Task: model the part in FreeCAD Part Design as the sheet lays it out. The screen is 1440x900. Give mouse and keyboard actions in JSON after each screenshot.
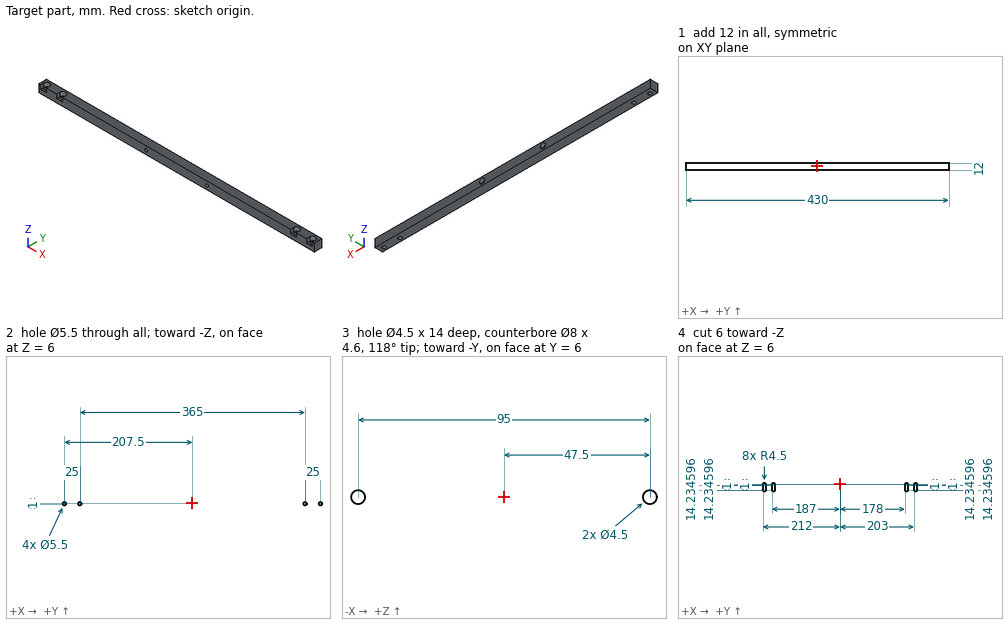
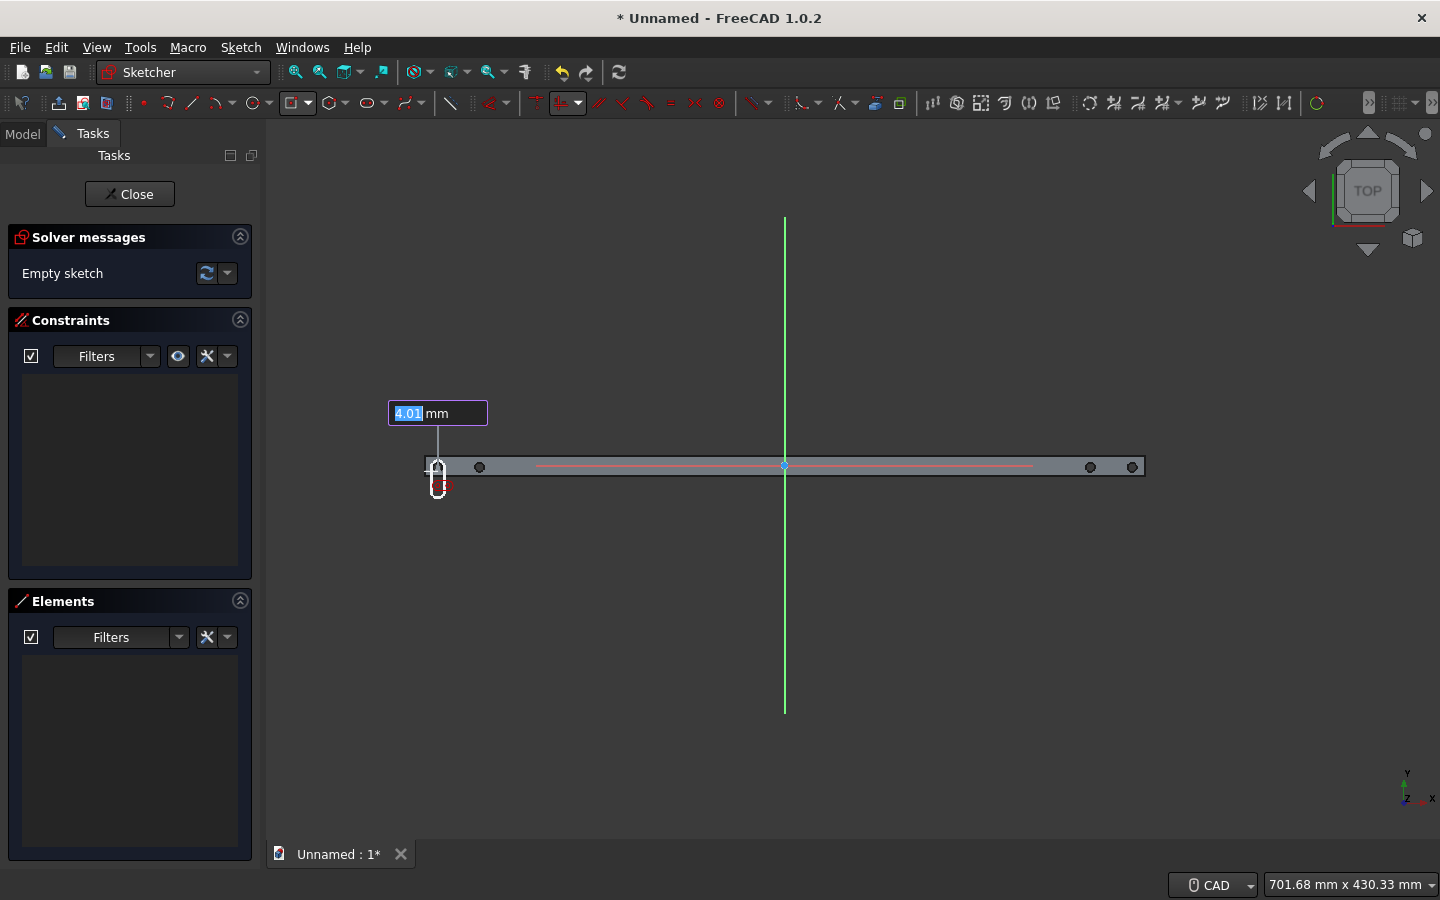
{"action": "scroll", "coordinate": [445, 479], "scroll_direction": "up", "scroll_amount": 4}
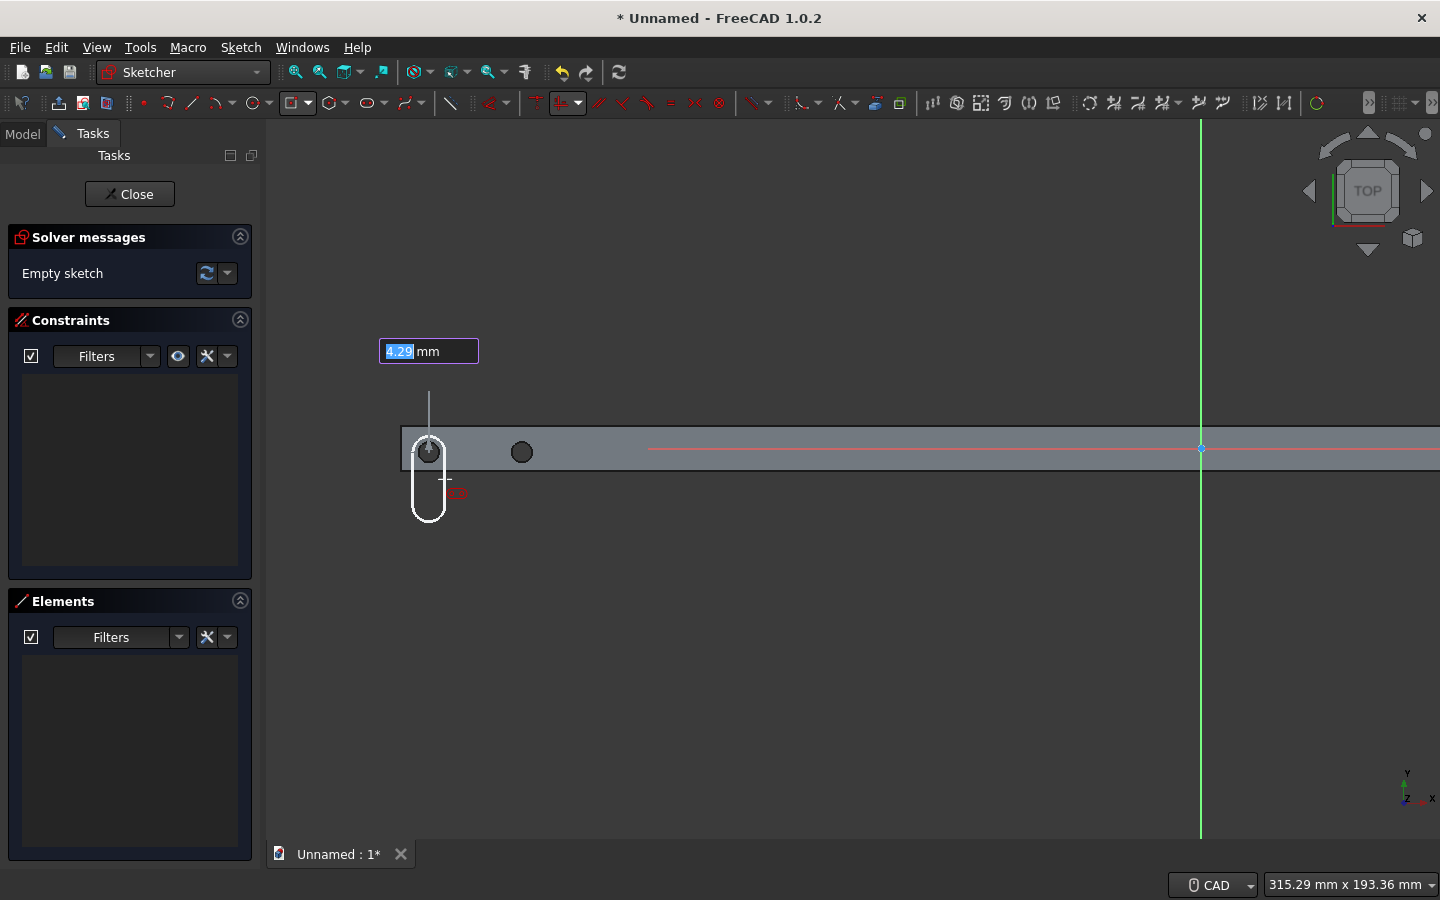
{"action": "left_click", "coordinate": [446, 479]}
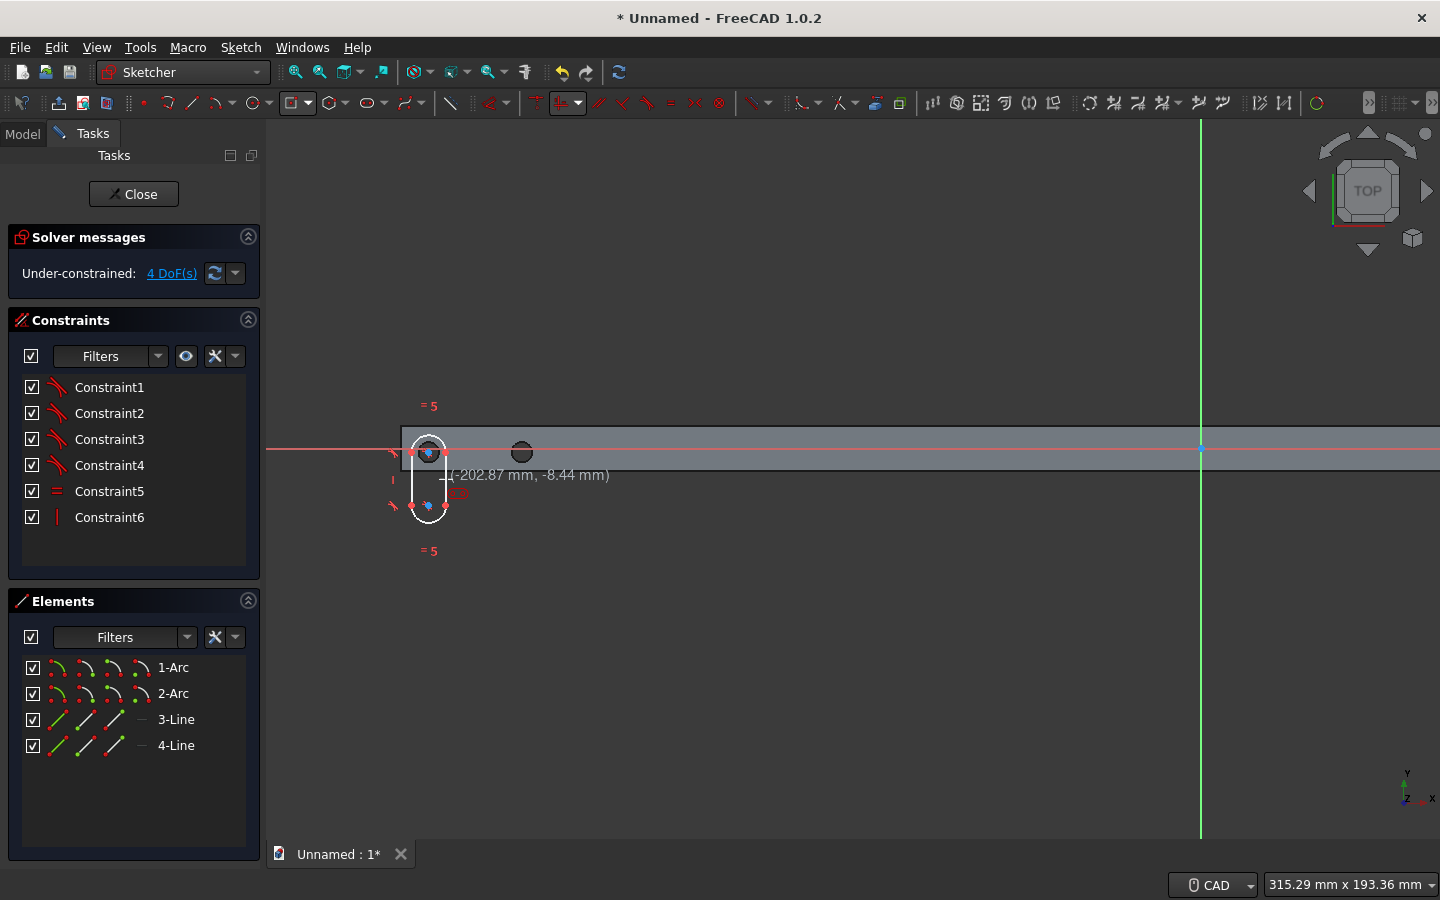
{"action": "scroll", "coordinate": [522, 505], "scroll_direction": "up", "scroll_amount": 2}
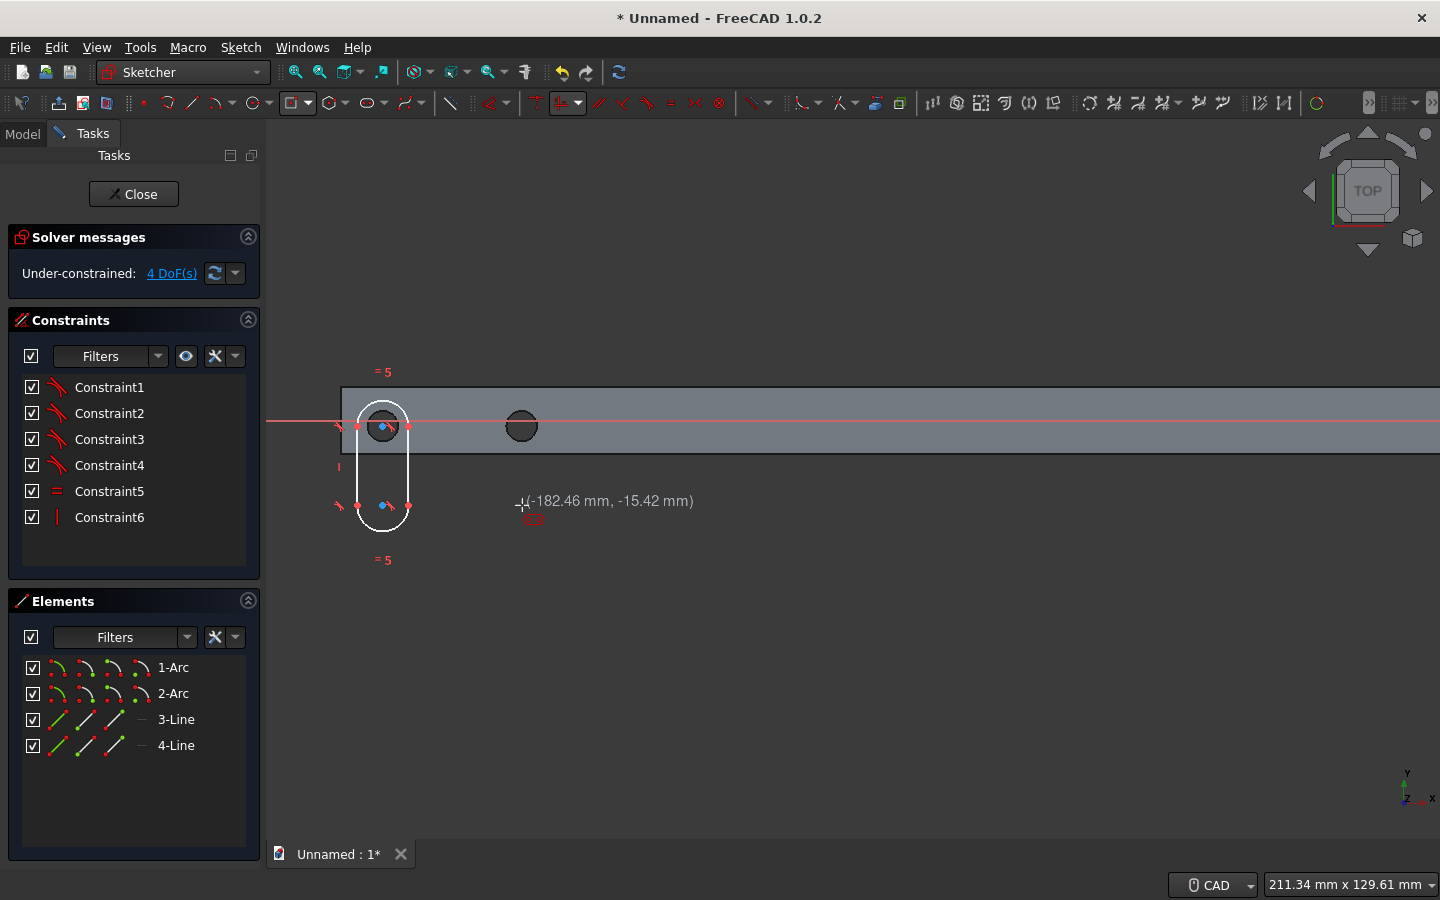
{"action": "left_click", "coordinate": [522, 505]}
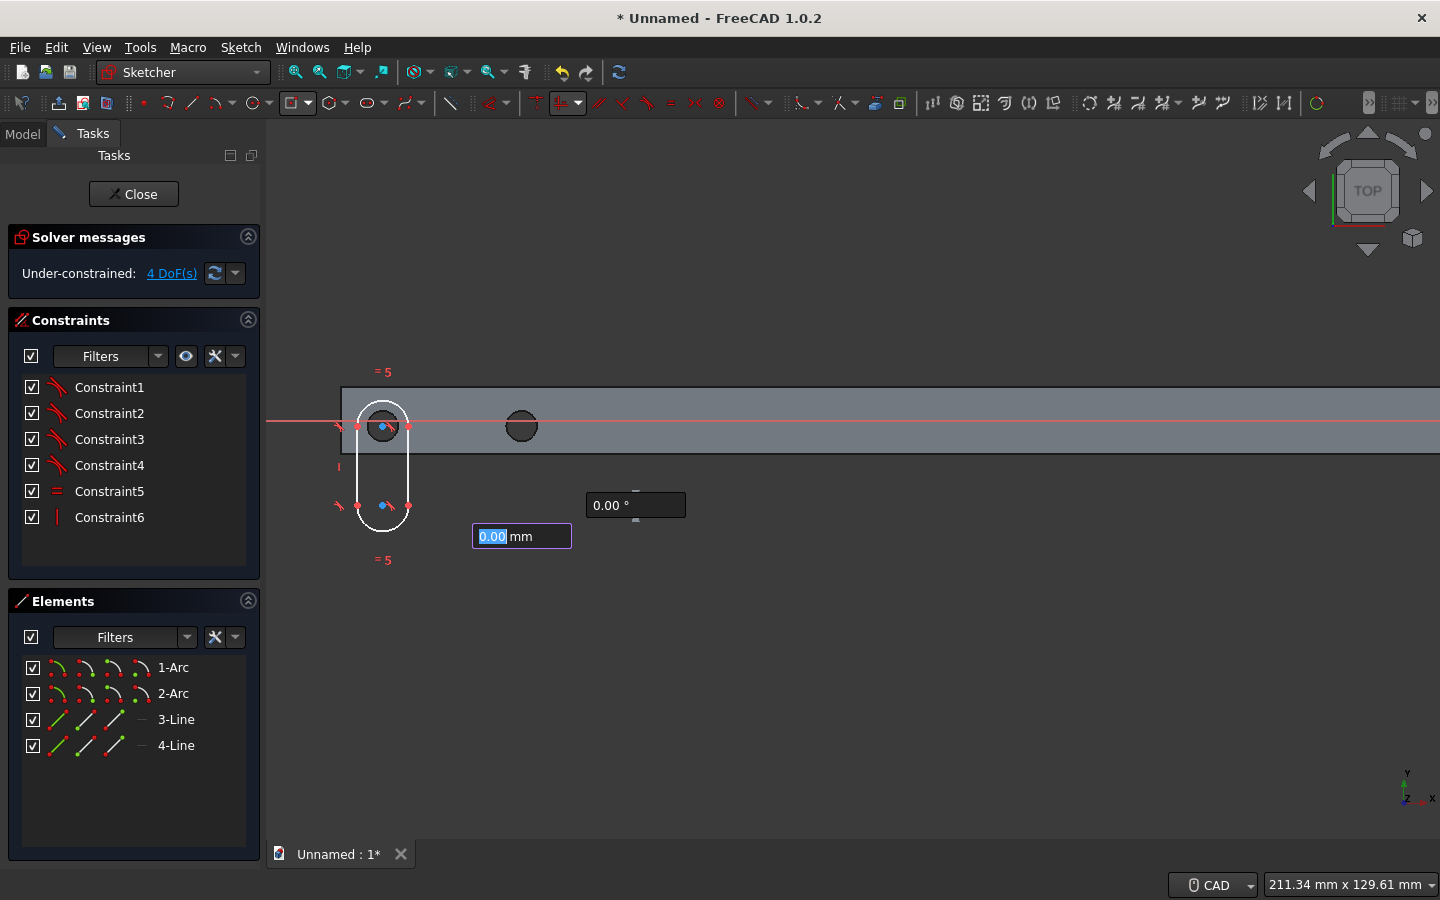
{"action": "scroll", "coordinate": [522, 426], "scroll_direction": "up", "scroll_amount": 6}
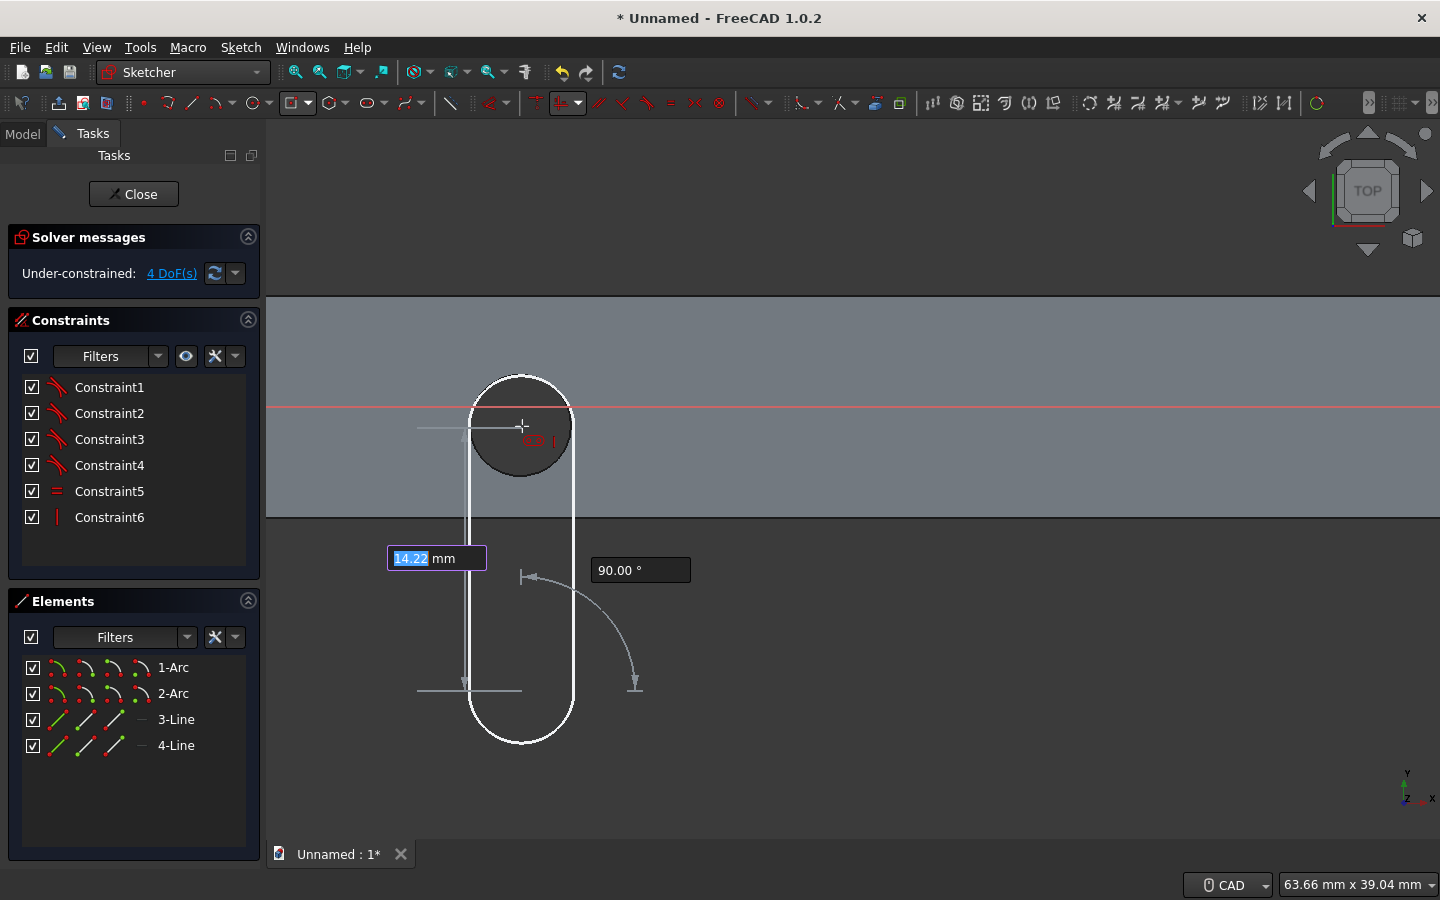
{"action": "left_click", "coordinate": [521, 425]}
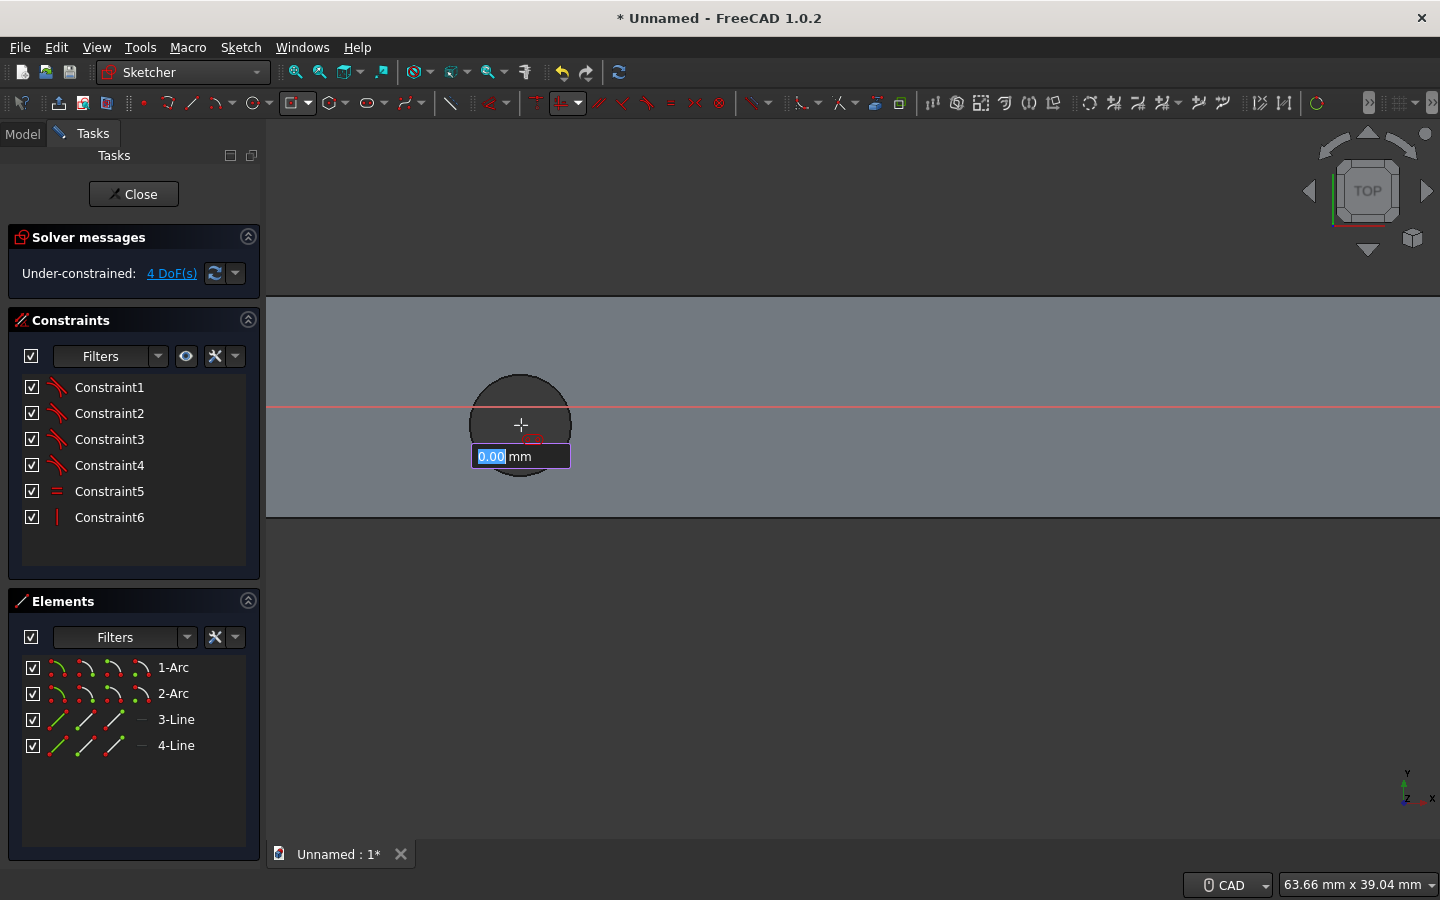
{"action": "scroll", "coordinate": [475, 471], "scroll_direction": "down", "scroll_amount": 12}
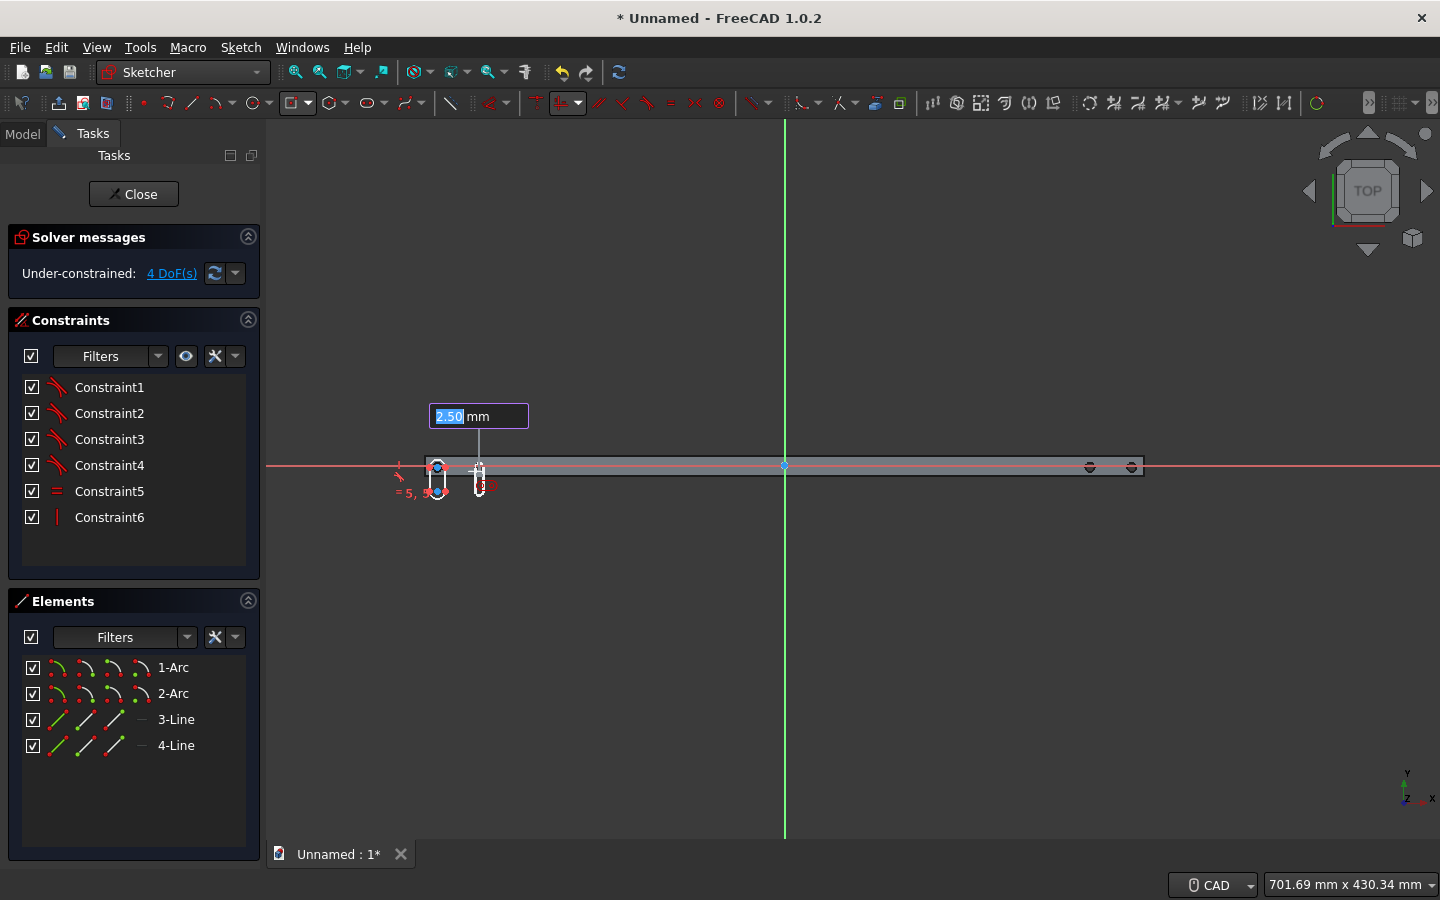
{"action": "scroll", "coordinate": [487, 479], "scroll_direction": "up", "scroll_amount": 4}